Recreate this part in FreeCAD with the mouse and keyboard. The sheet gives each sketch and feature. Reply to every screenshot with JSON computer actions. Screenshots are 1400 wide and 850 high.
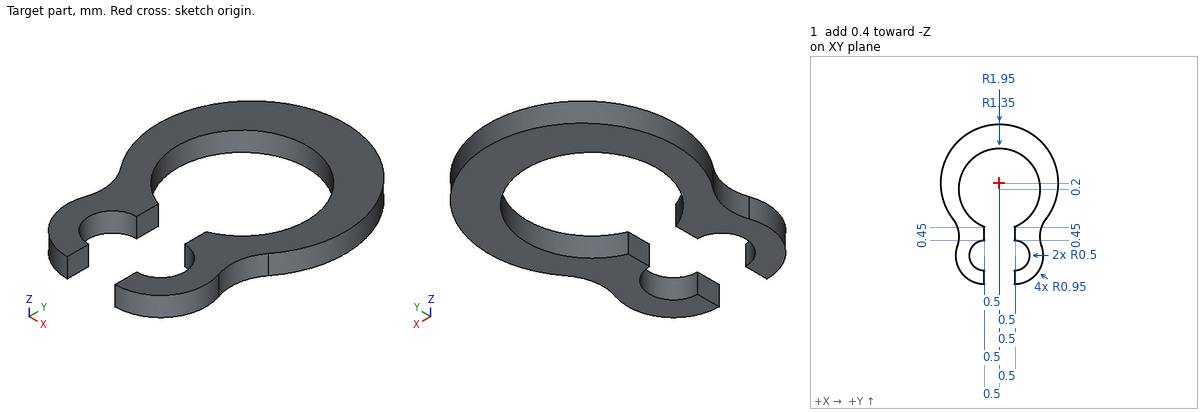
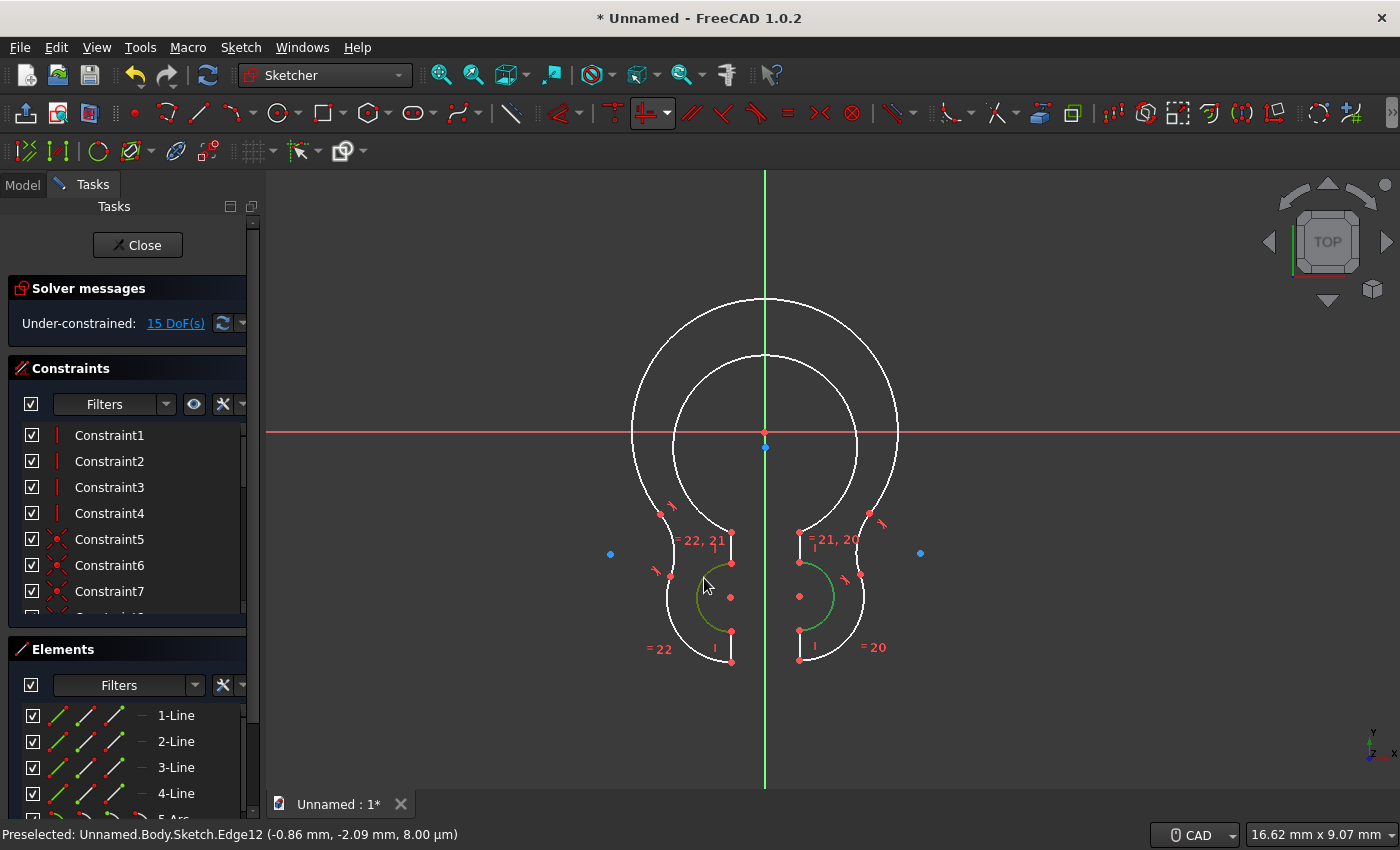
{"action": "left_click", "coordinate": [788, 114]}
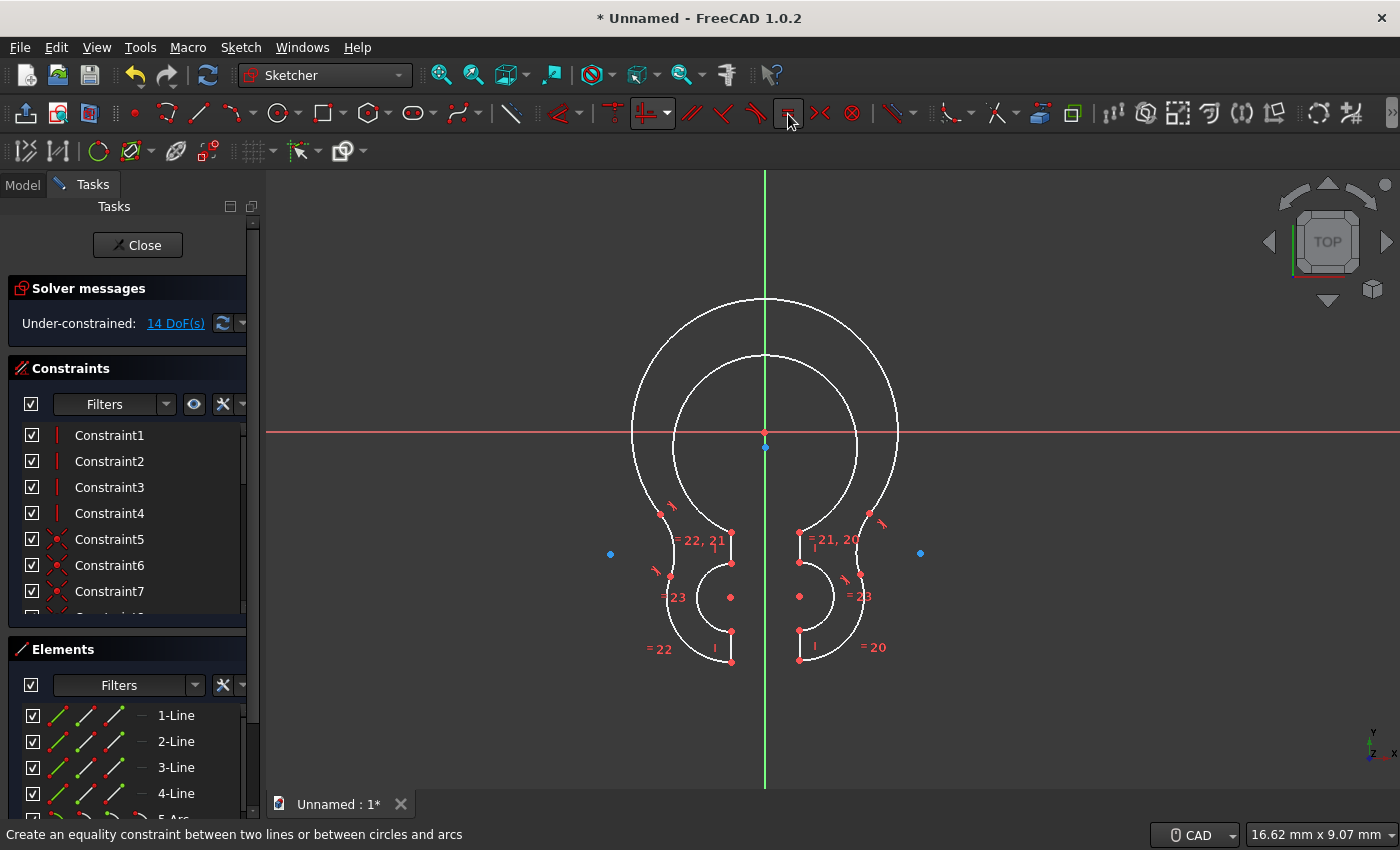
{"action": "left_click", "coordinate": [765, 447]}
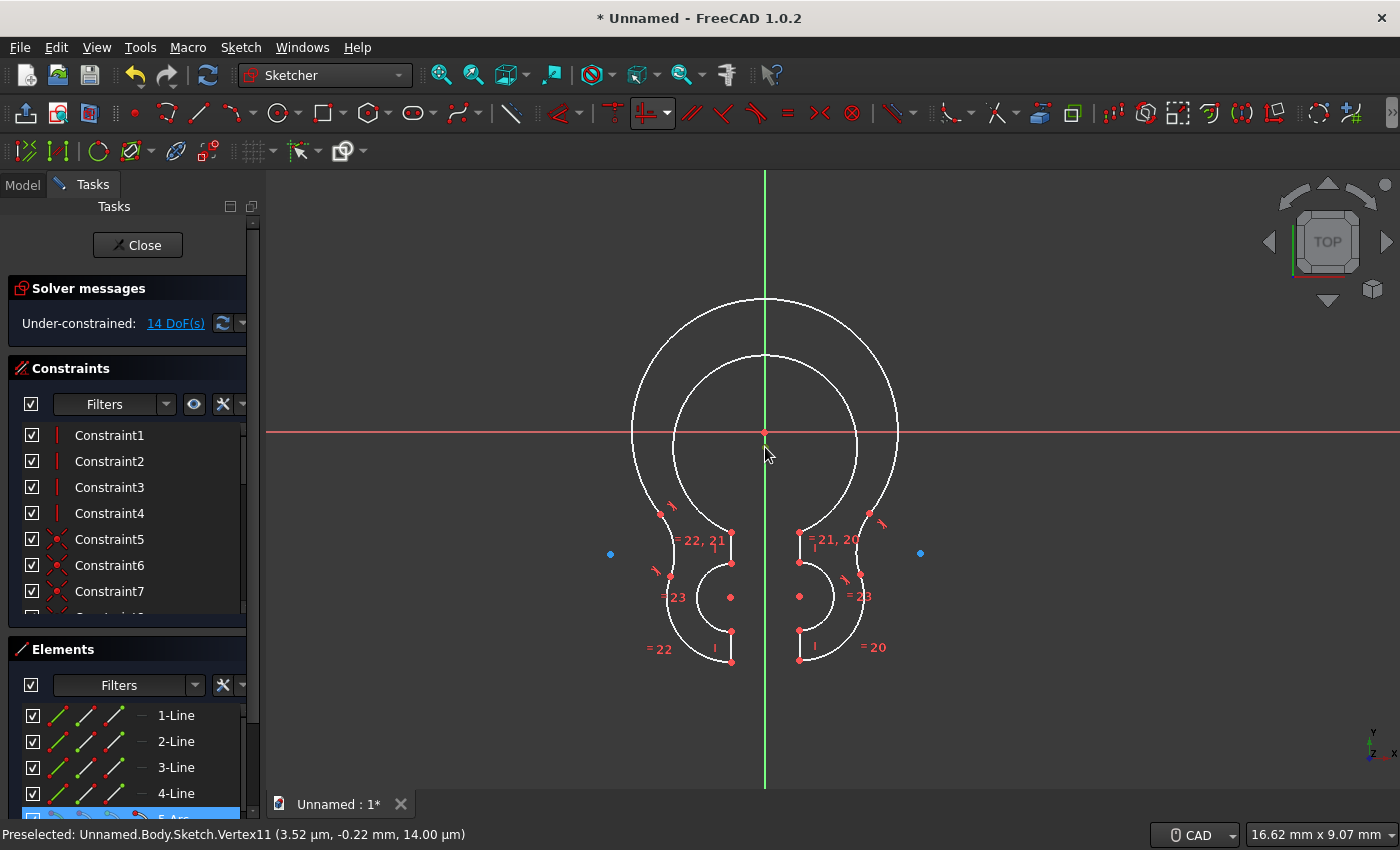
{"action": "left_click", "coordinate": [765, 721]}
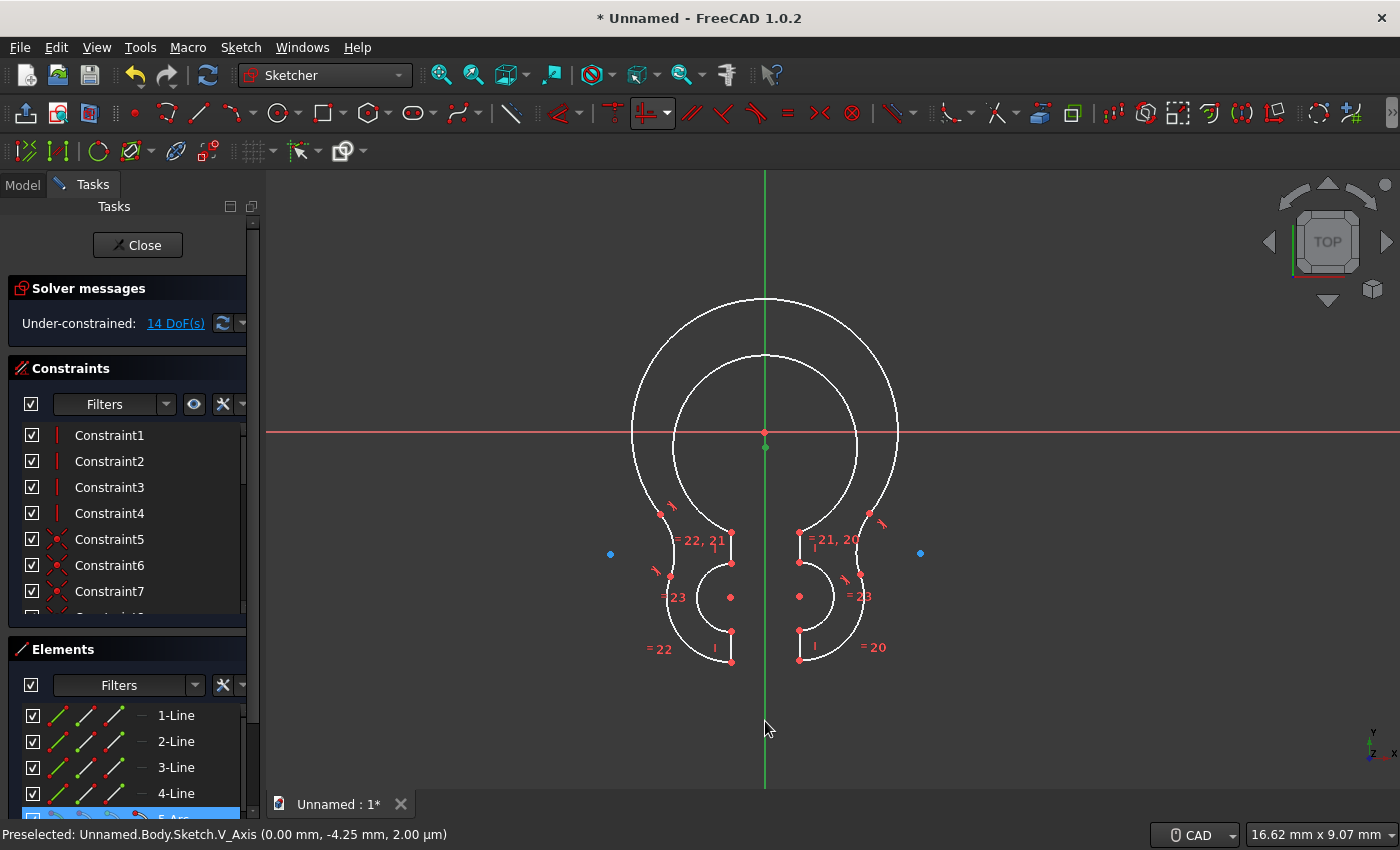
{"action": "left_click", "coordinate": [614, 114]}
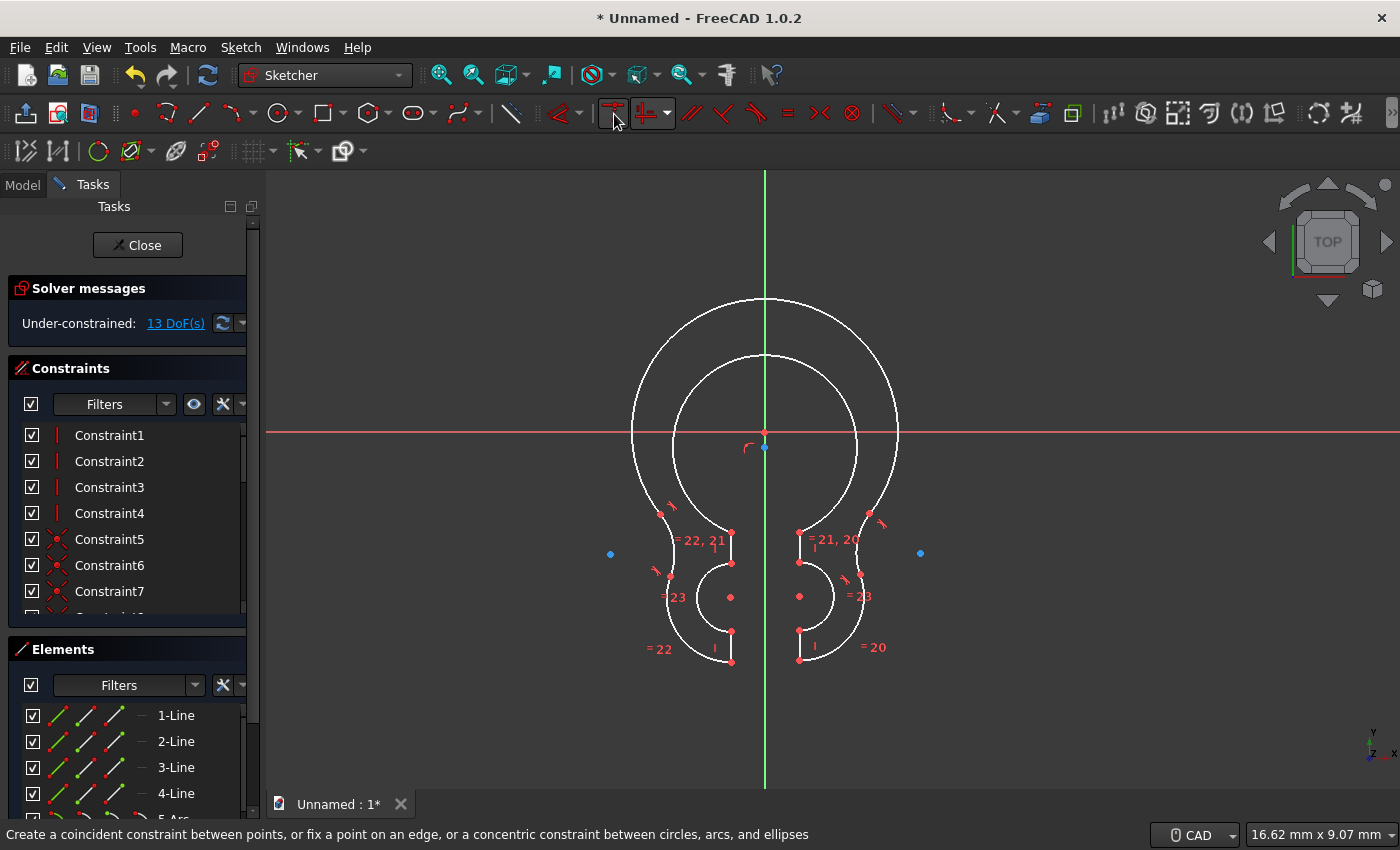
{"action": "left_click", "coordinate": [558, 114]}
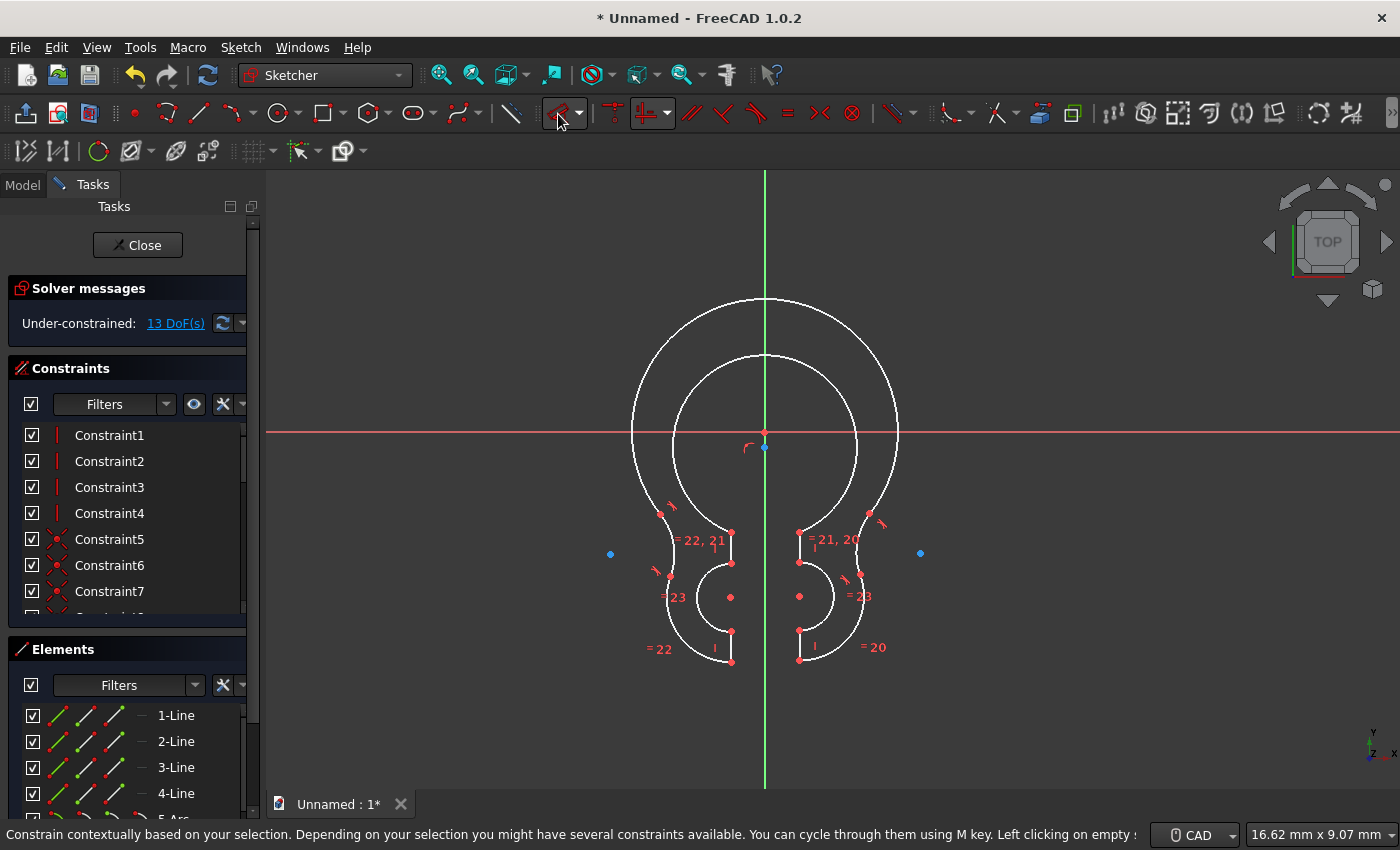
{"action": "left_click", "coordinate": [847, 405]}
{"action": "left_click", "coordinate": [875, 390]}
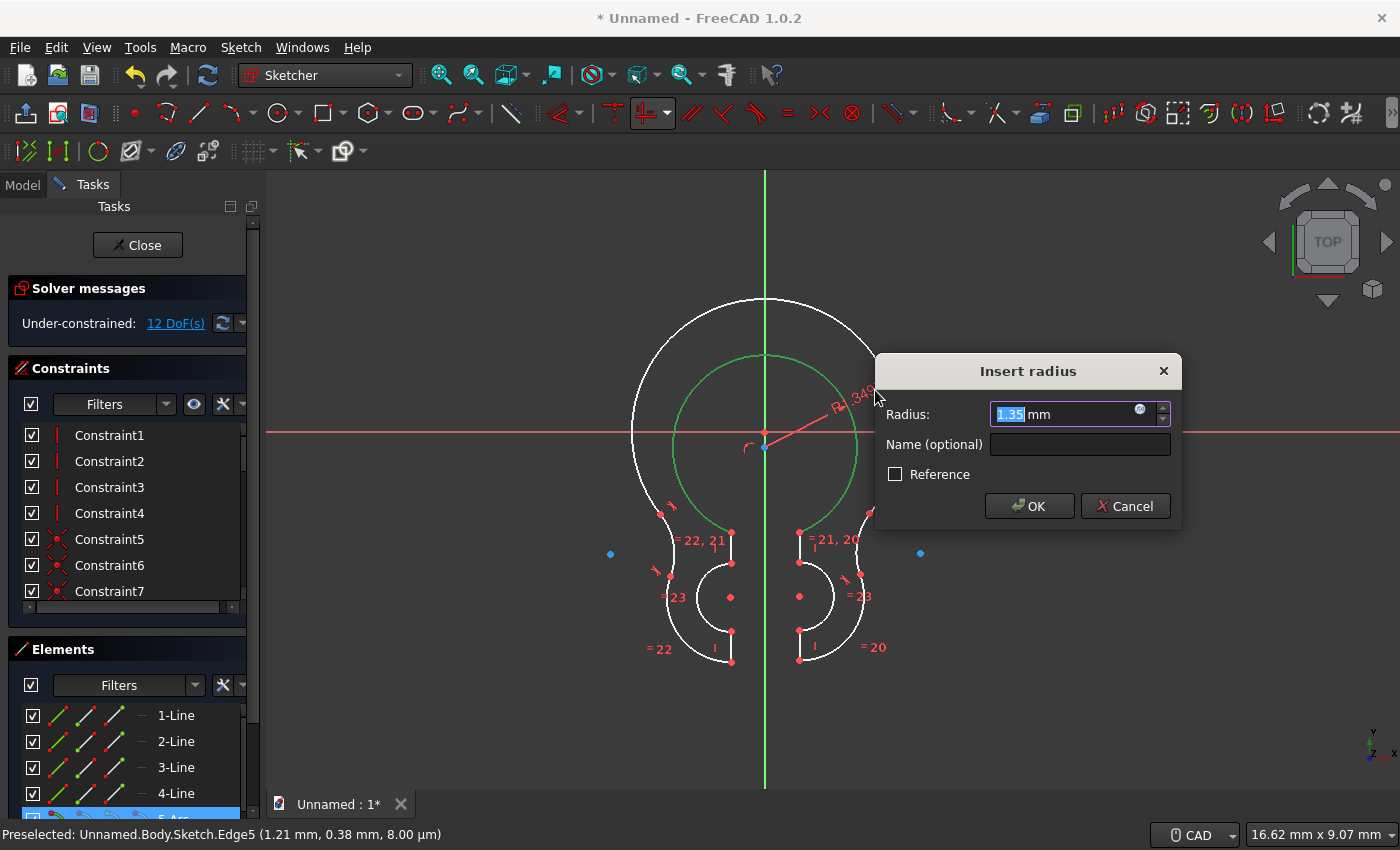
{"action": "type", "text": "1.35"}
{"action": "key", "text": "Return"}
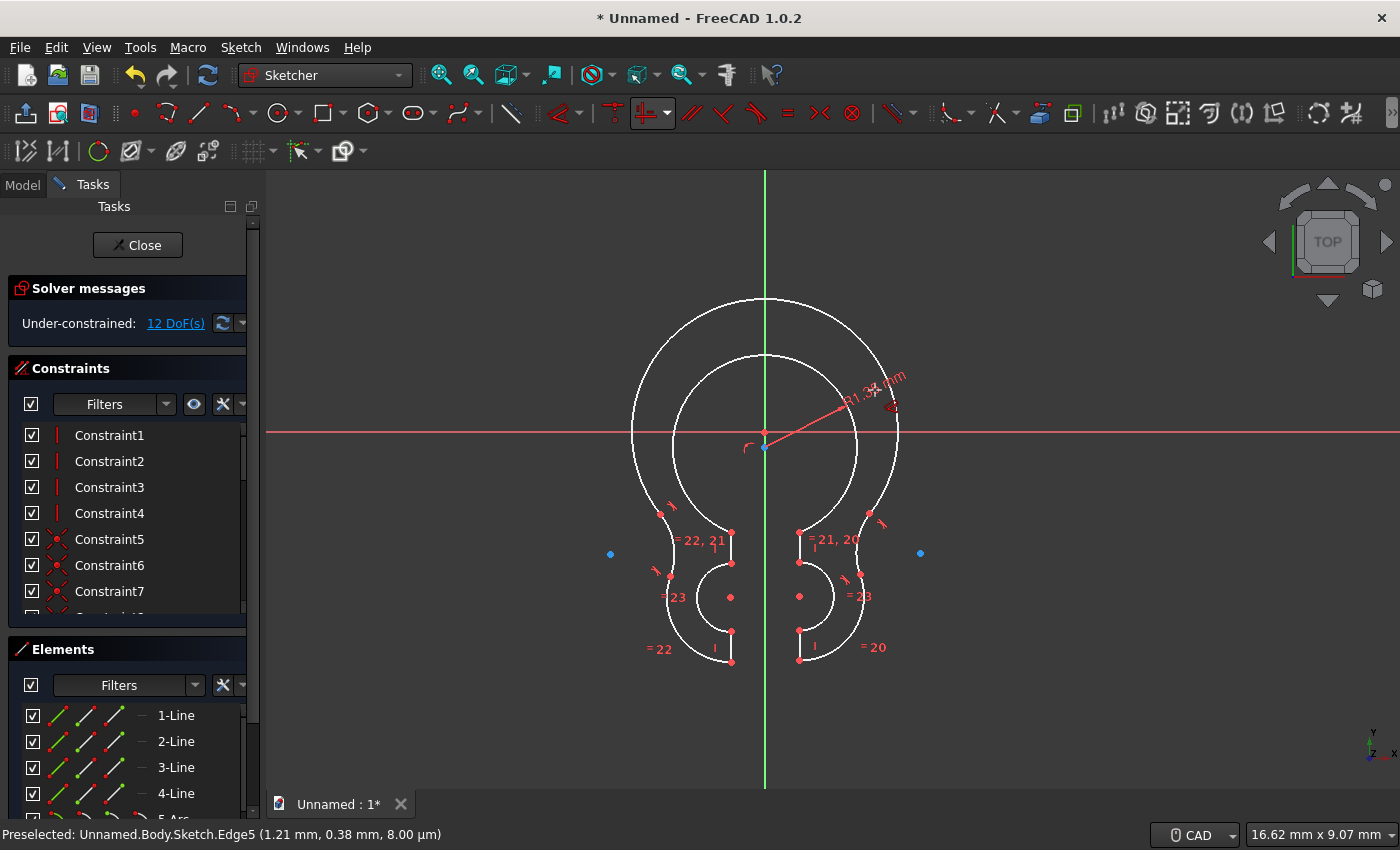
{"action": "left_click", "coordinate": [827, 616]}
{"action": "left_click", "coordinate": [838, 543]}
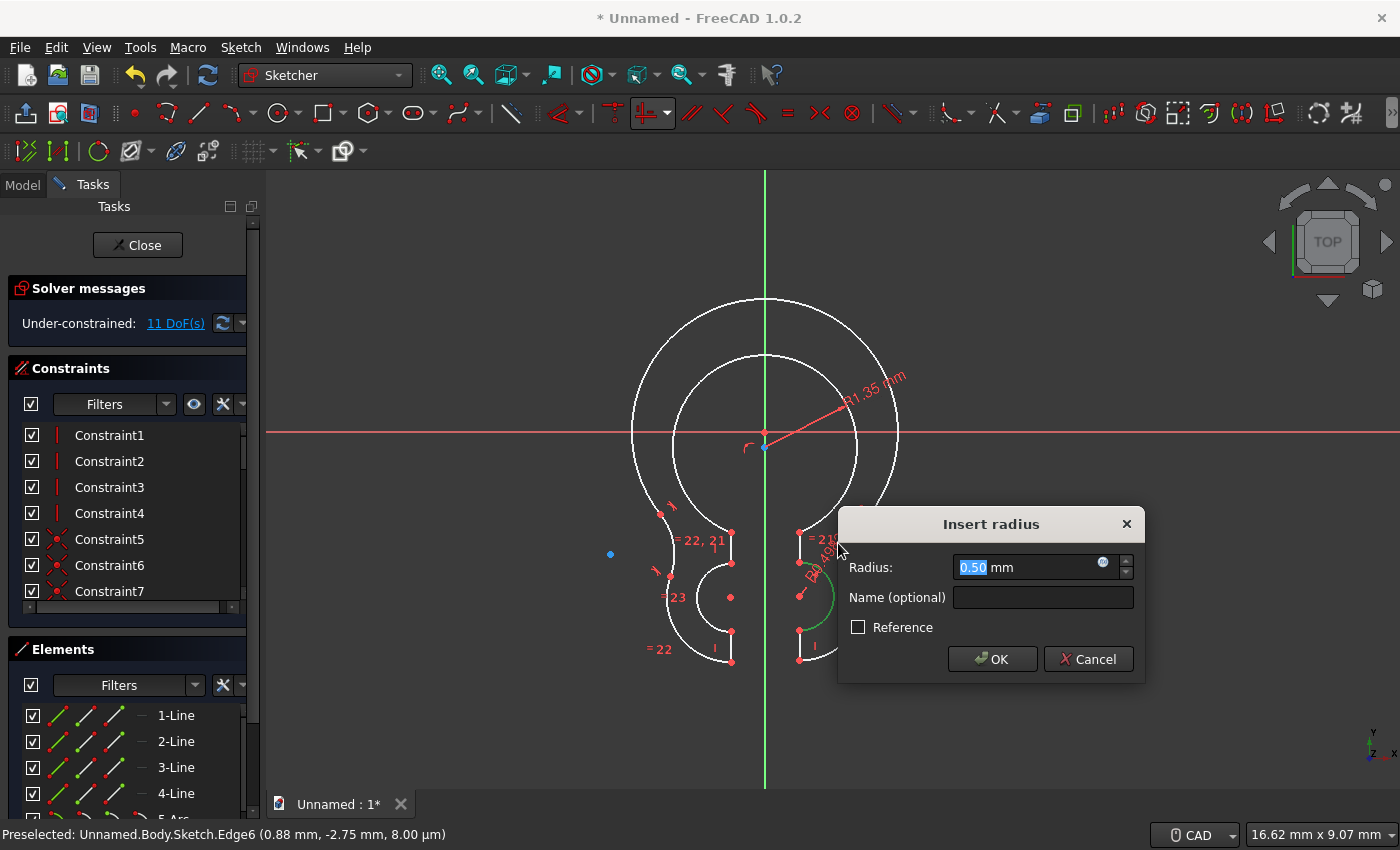
{"action": "type", "text": "0.5"}
{"action": "key", "text": "Return"}